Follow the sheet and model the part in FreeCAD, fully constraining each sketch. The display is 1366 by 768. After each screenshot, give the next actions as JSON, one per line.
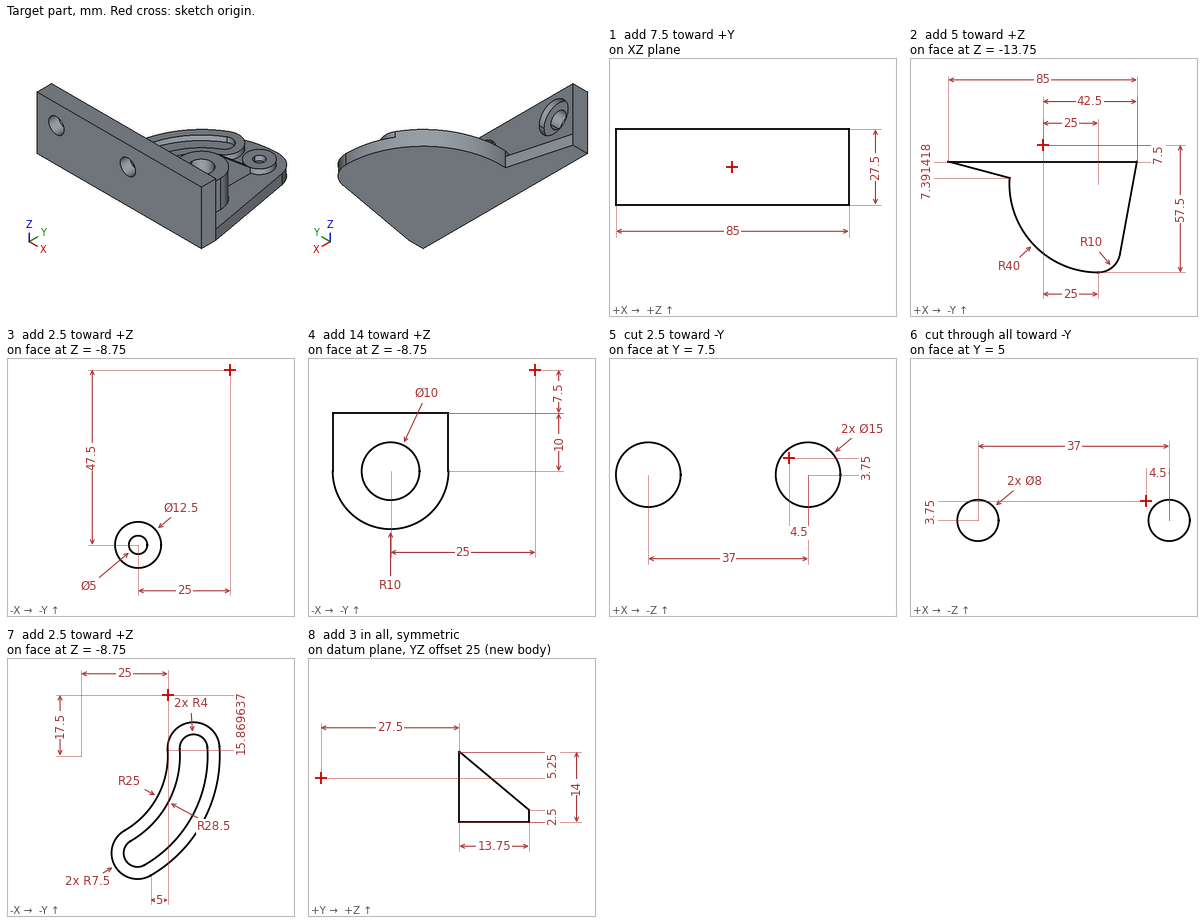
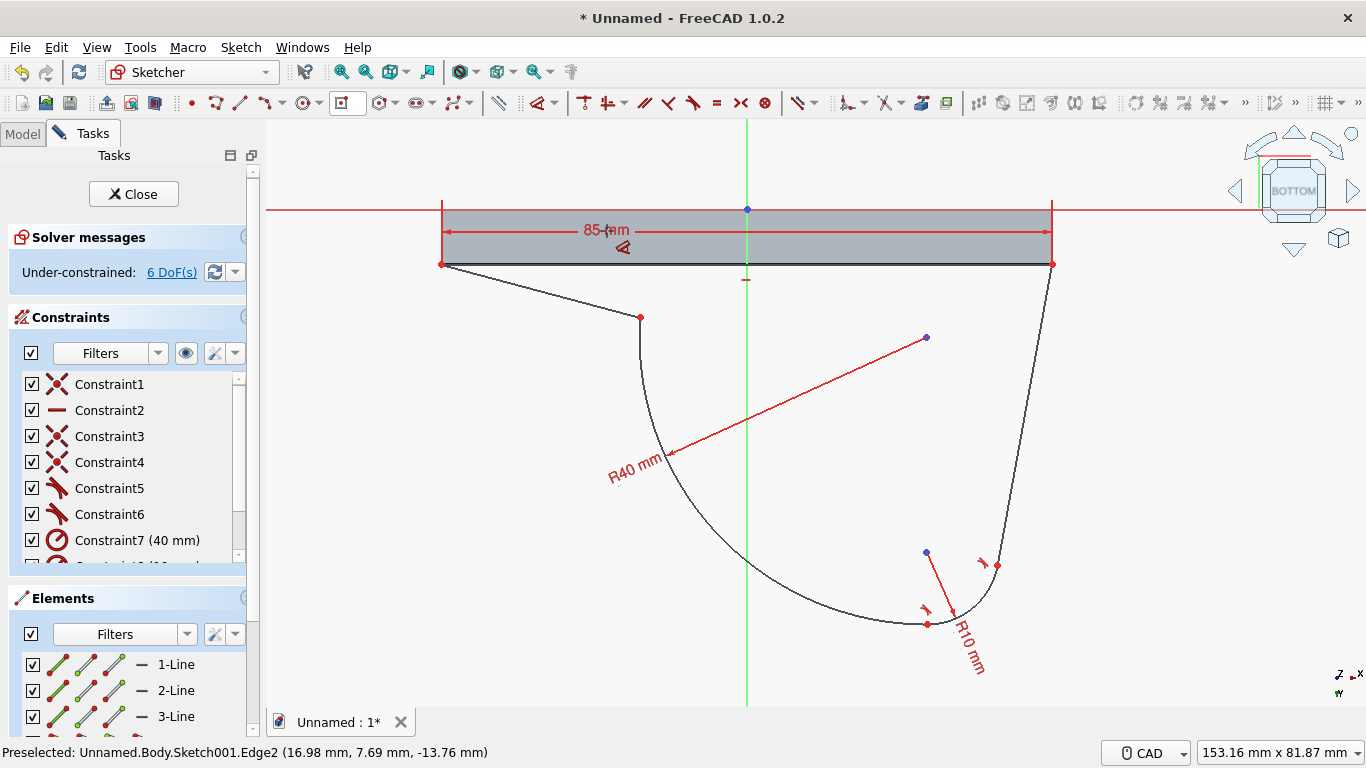
{"action": "left_click", "coordinate": [927, 625]}
{"action": "left_click", "coordinate": [837, 659]}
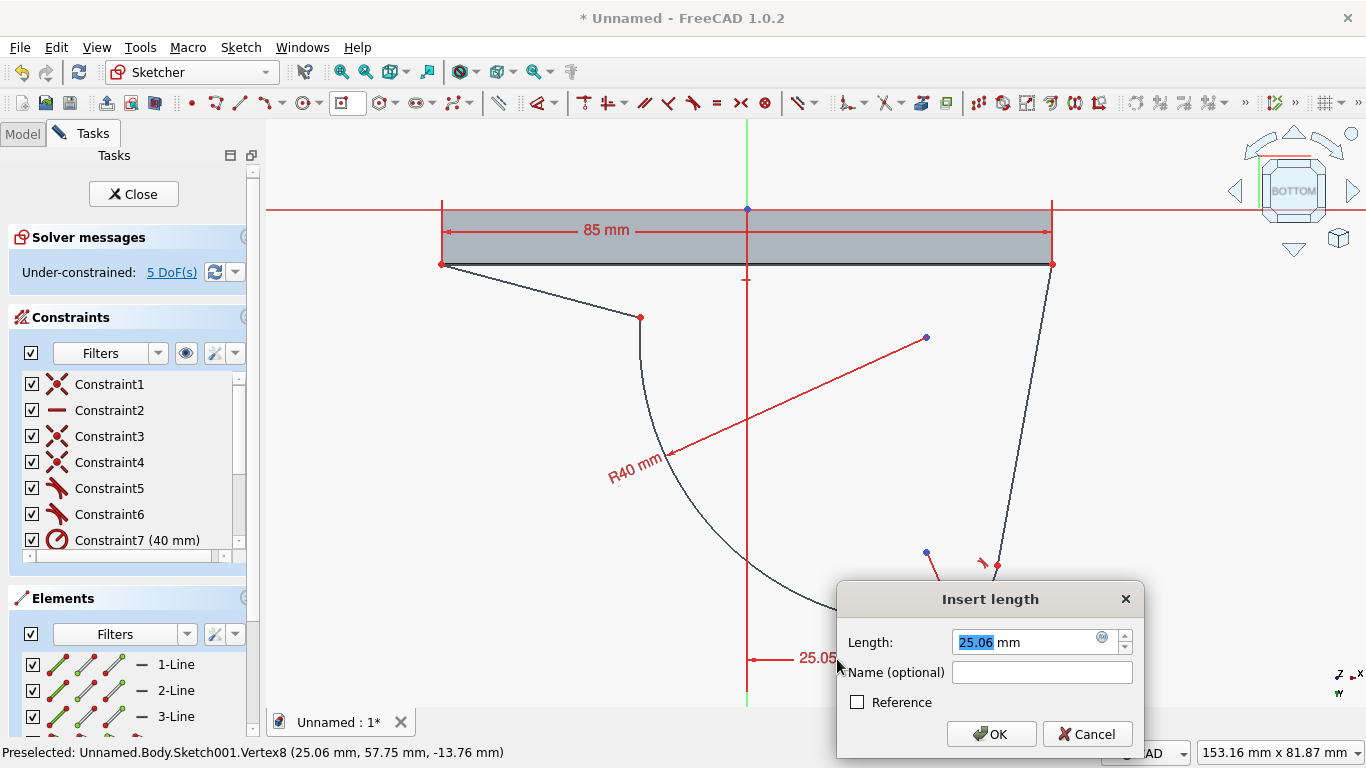
{"action": "type", "text": "25"}
{"action": "key", "text": "Return"}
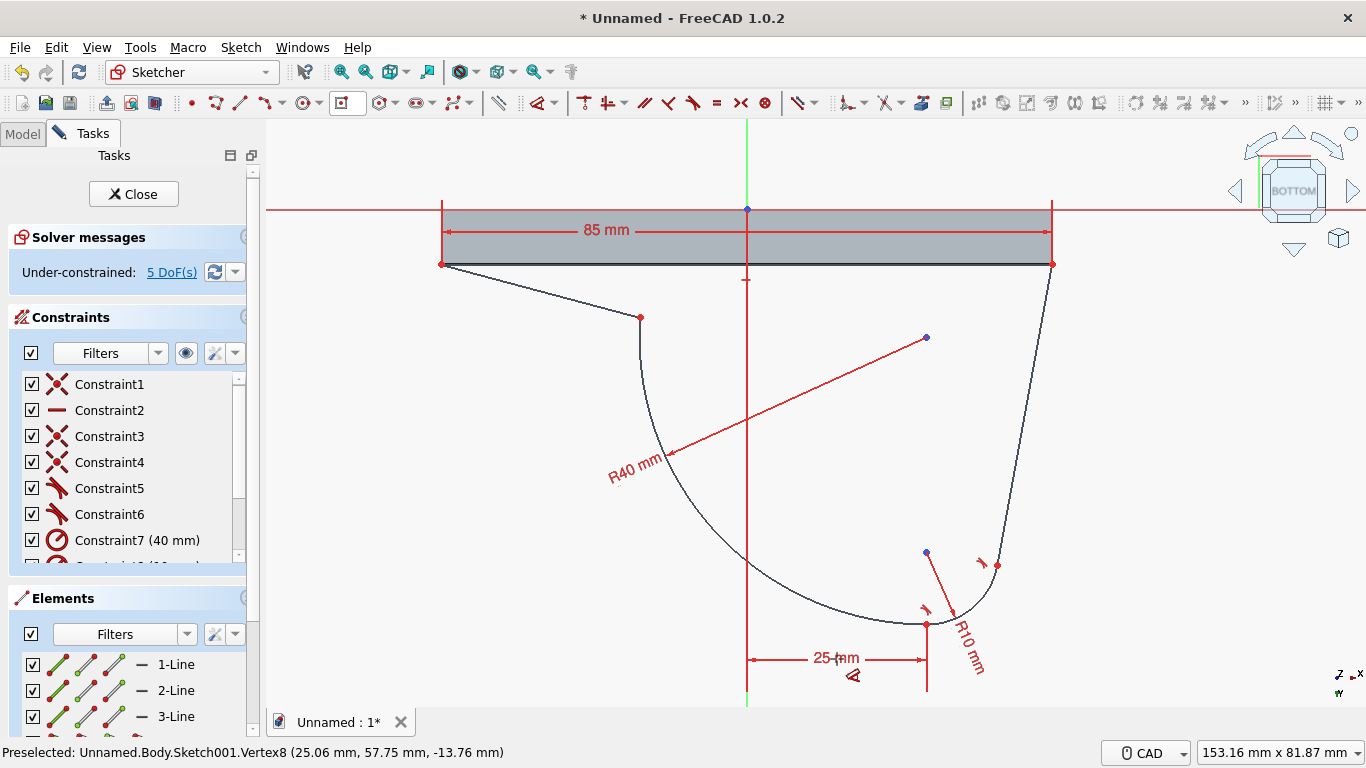
{"action": "left_click", "coordinate": [927, 337]}
{"action": "left_click", "coordinate": [837, 176]}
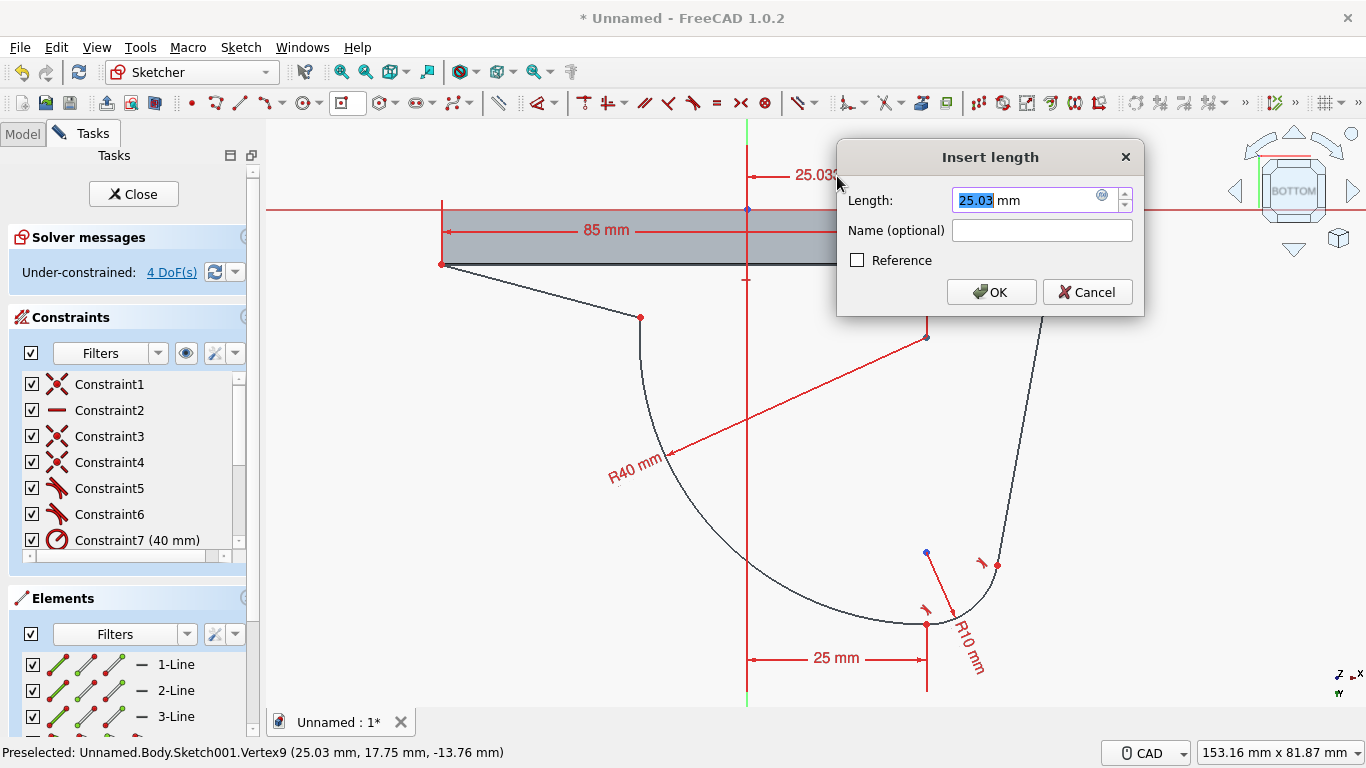
{"action": "type", "text": "25"}
{"action": "key", "text": "Return"}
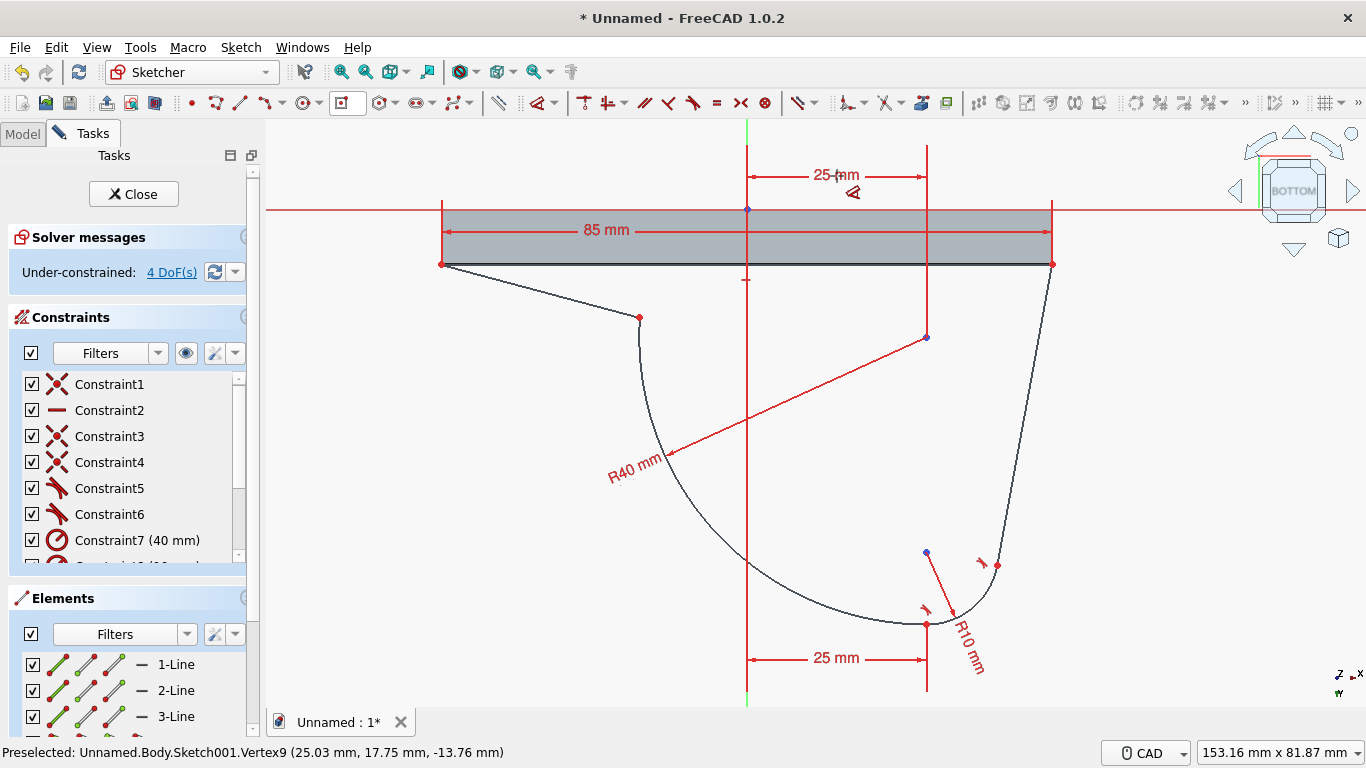
{"action": "left_click", "coordinate": [1052, 265]}
{"action": "left_click", "coordinate": [1086, 237]}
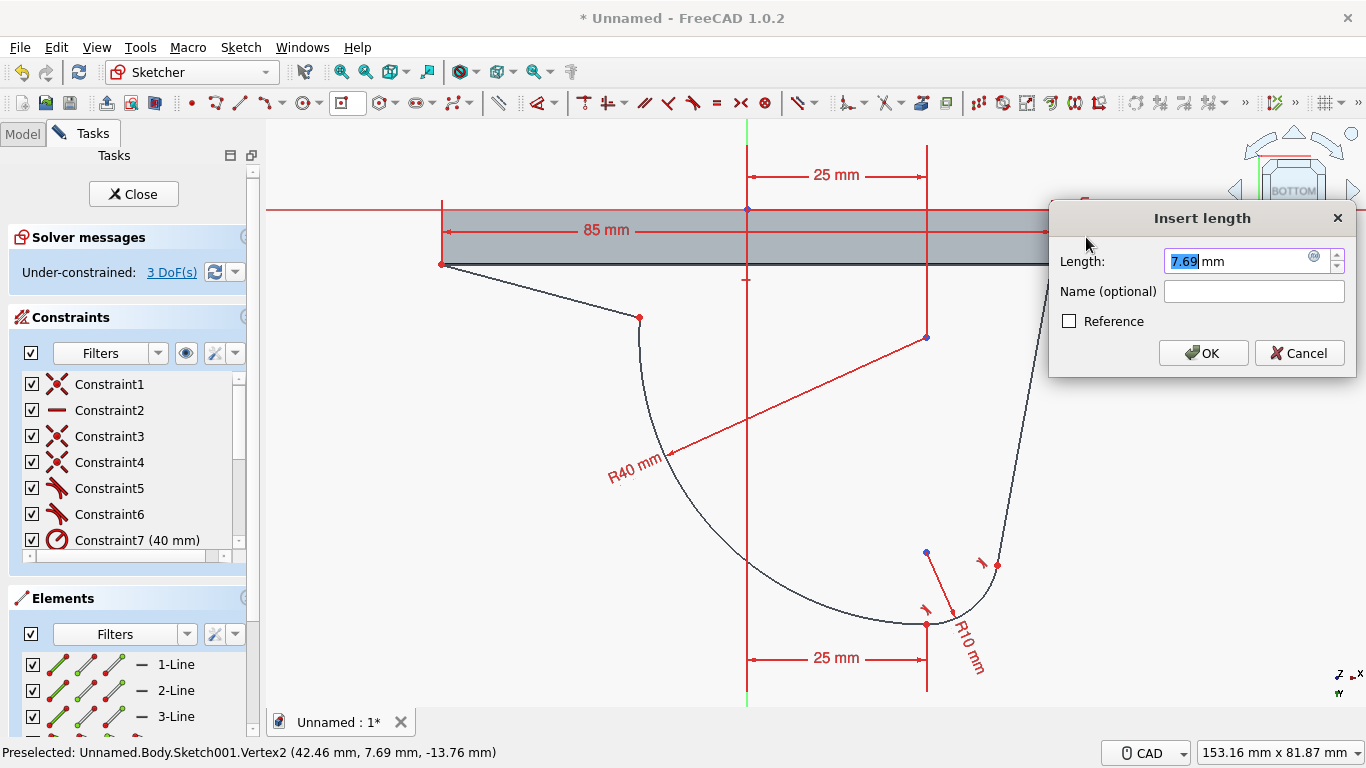
{"action": "type", "text": "7.5"}
{"action": "key", "text": "Return"}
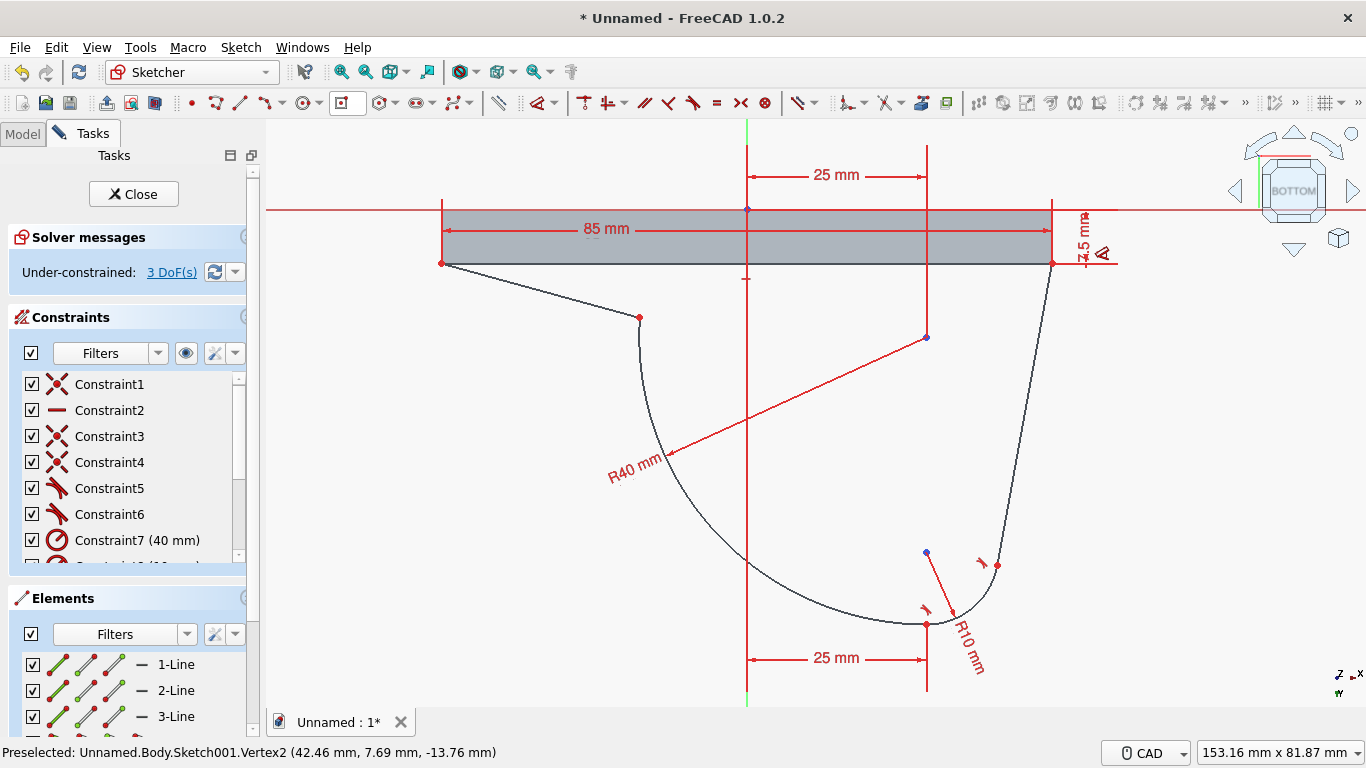
{"action": "left_click", "coordinate": [1052, 264]}
{"action": "left_click", "coordinate": [970, 176]}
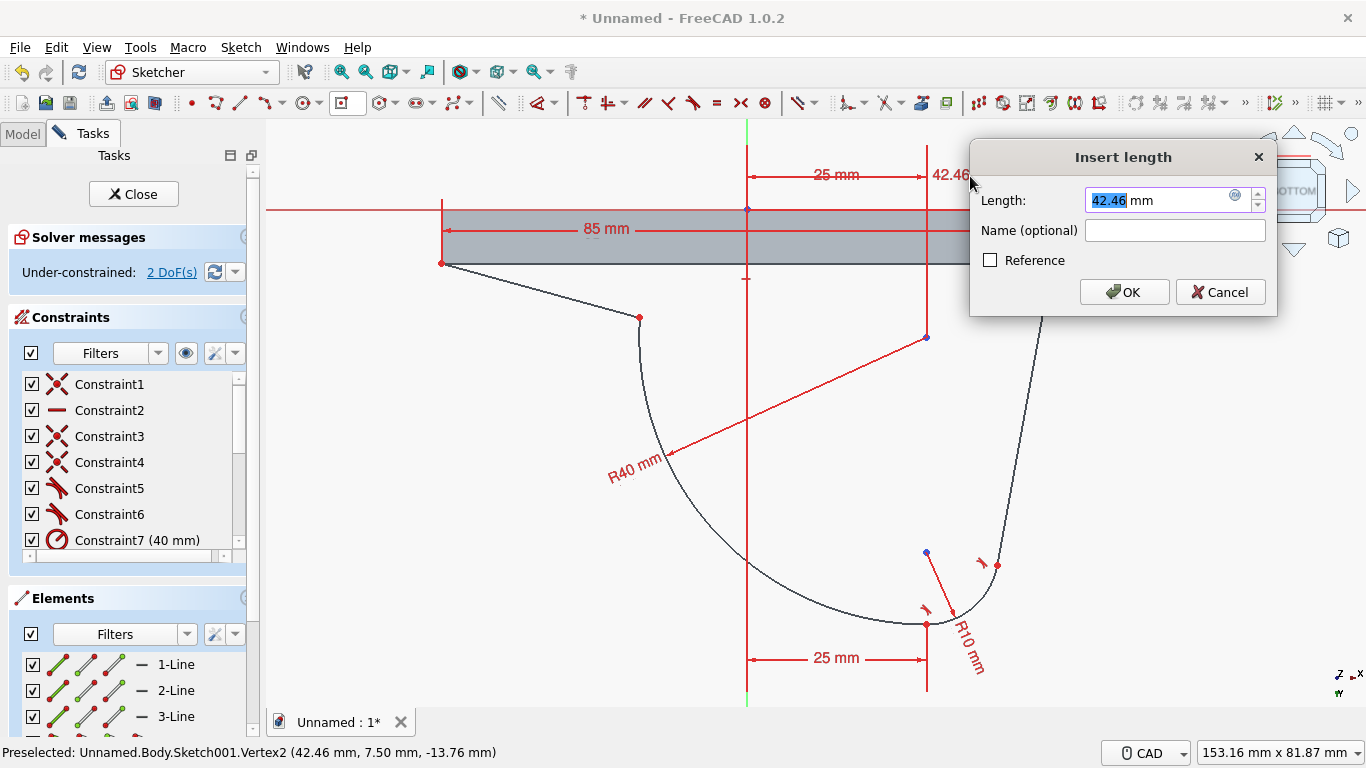
{"action": "type", "text": "42.5"}
{"action": "key", "text": "Return"}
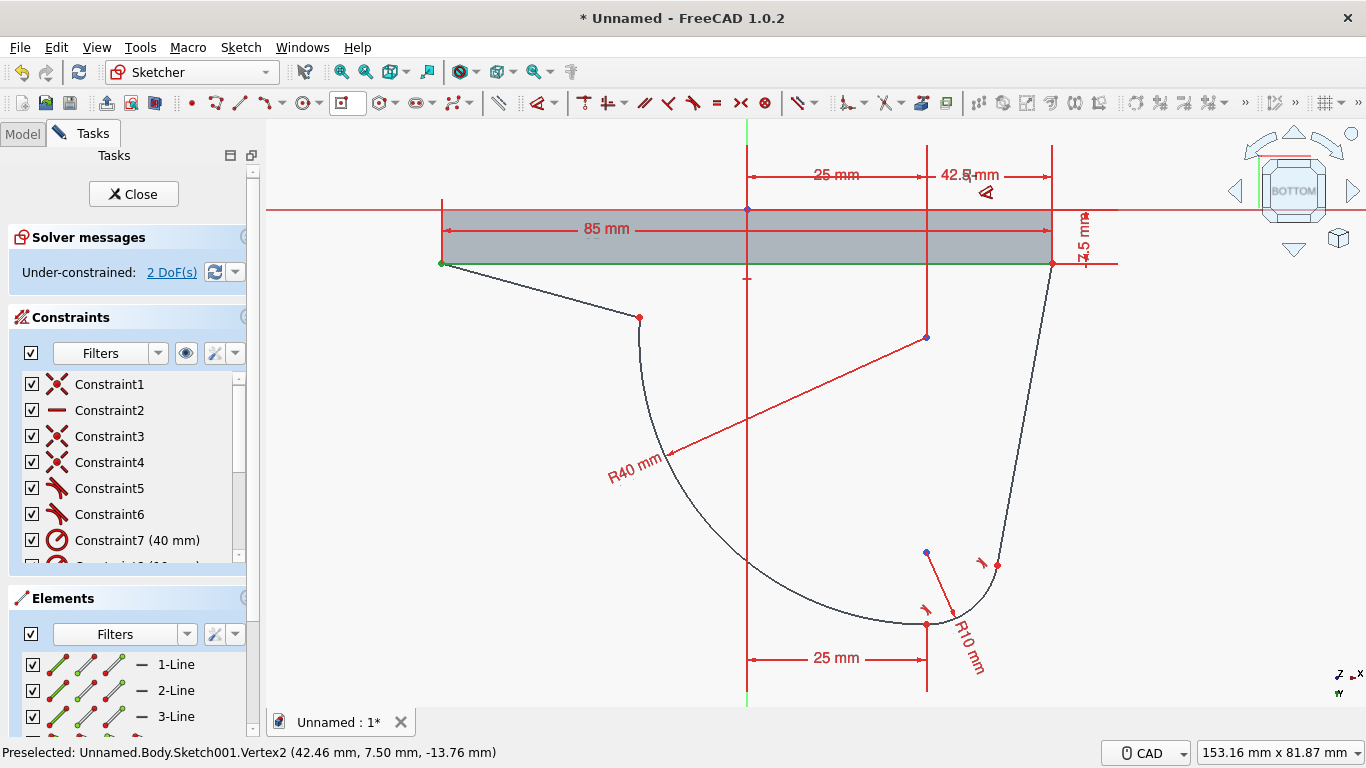
{"action": "left_click", "coordinate": [927, 625]}
{"action": "left_click", "coordinate": [961, 417]}